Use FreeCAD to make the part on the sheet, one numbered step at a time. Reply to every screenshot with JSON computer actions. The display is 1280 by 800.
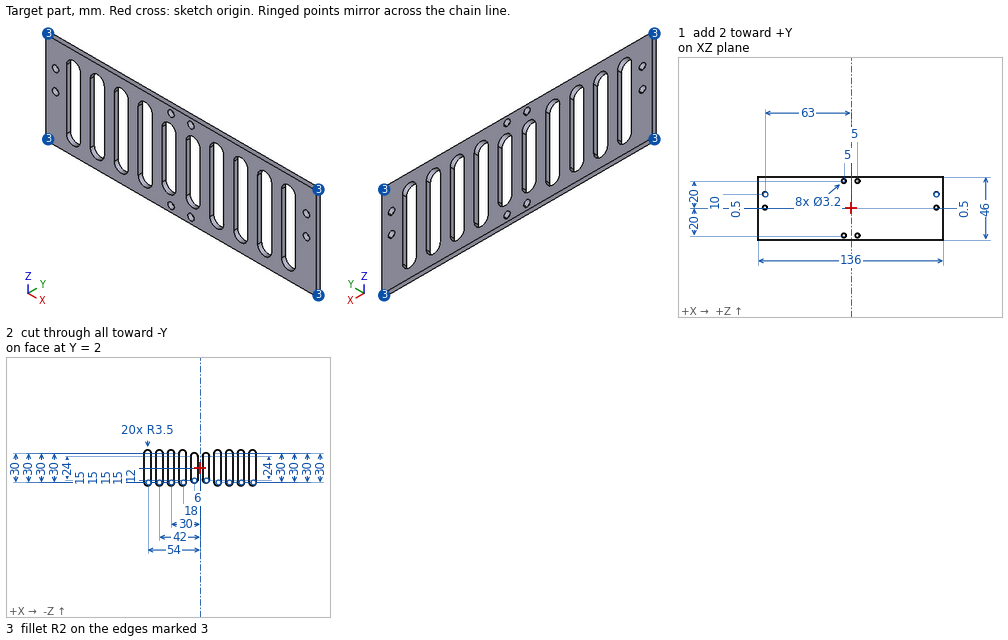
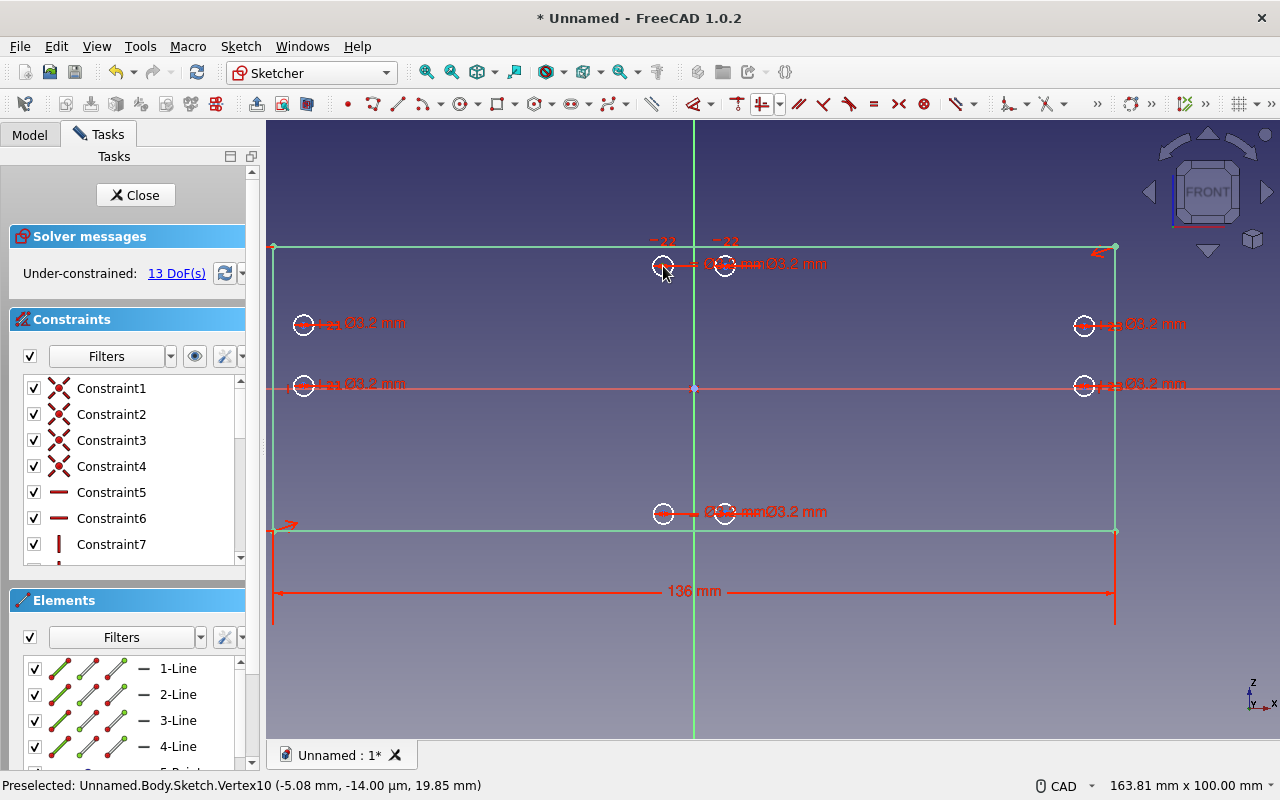
{"action": "left_click", "coordinate": [663, 514]}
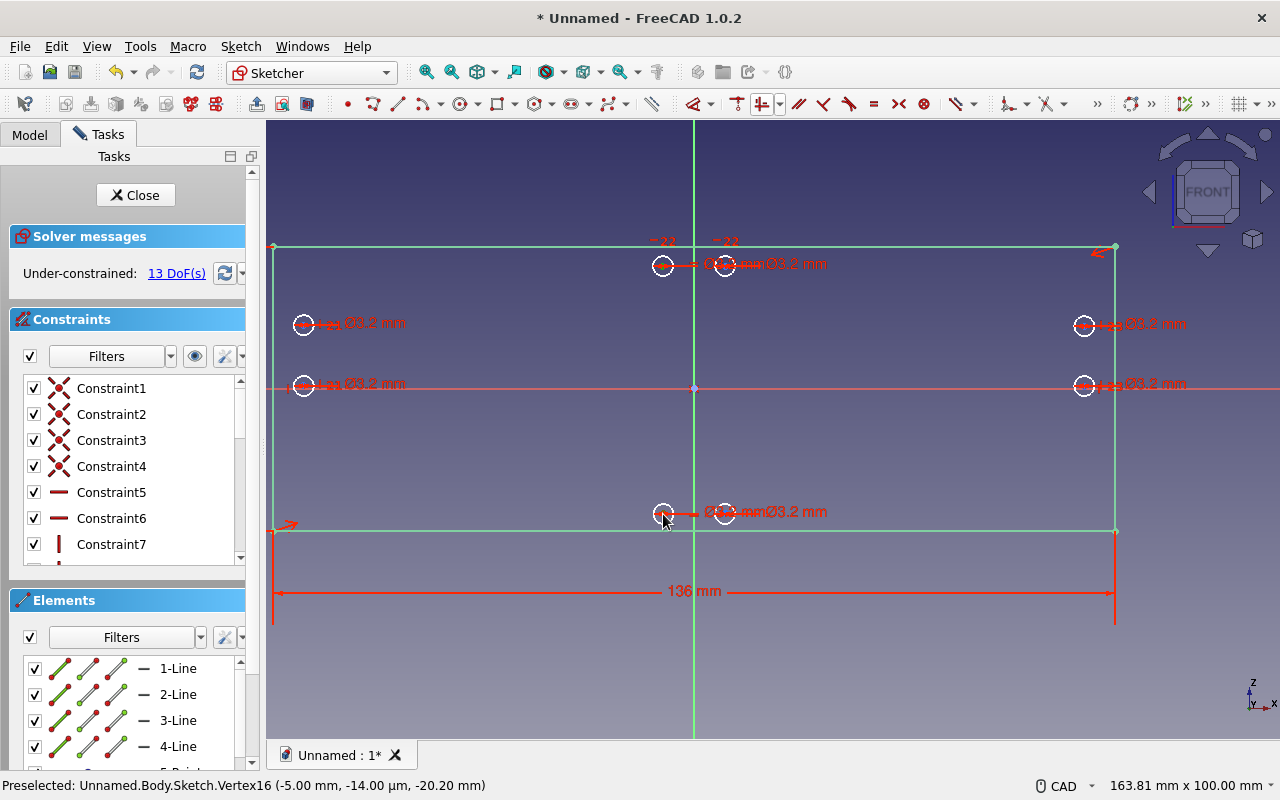
{"action": "left_click", "coordinate": [780, 104]}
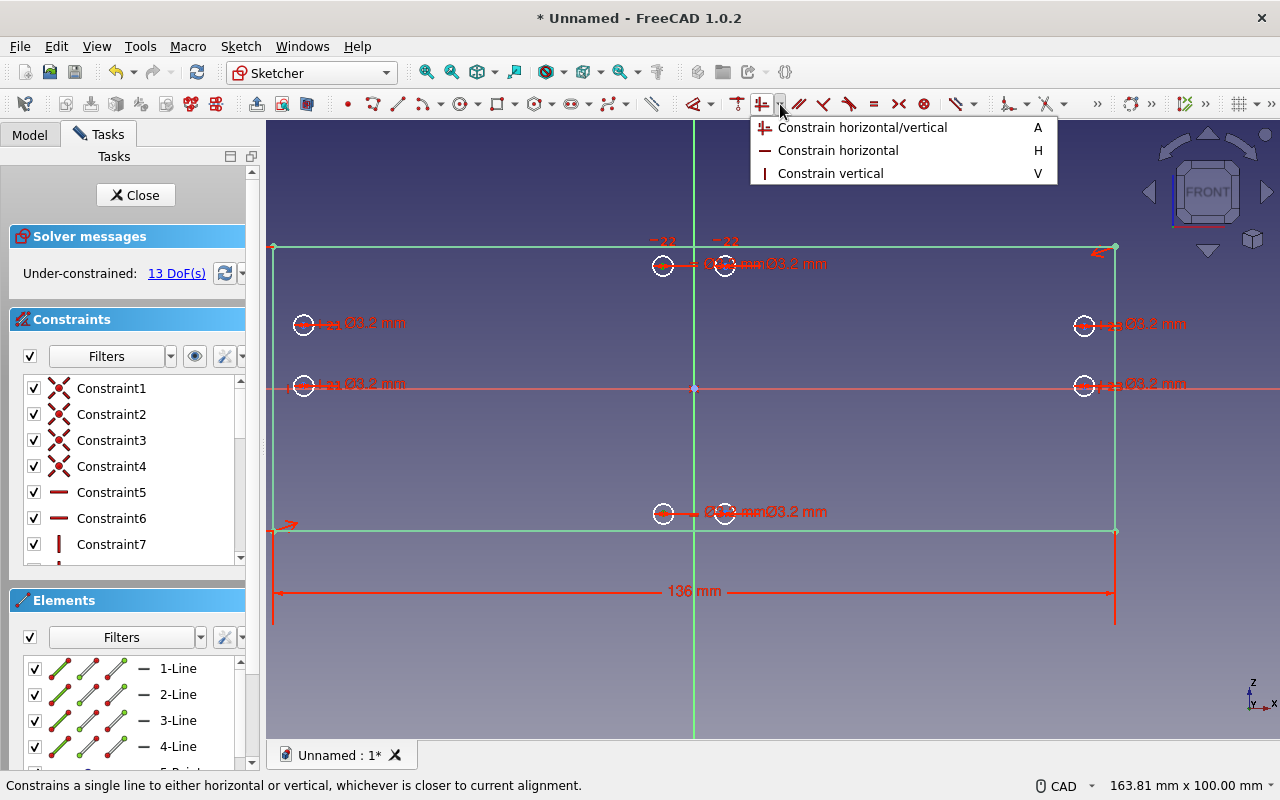
{"action": "left_click", "coordinate": [904, 174]}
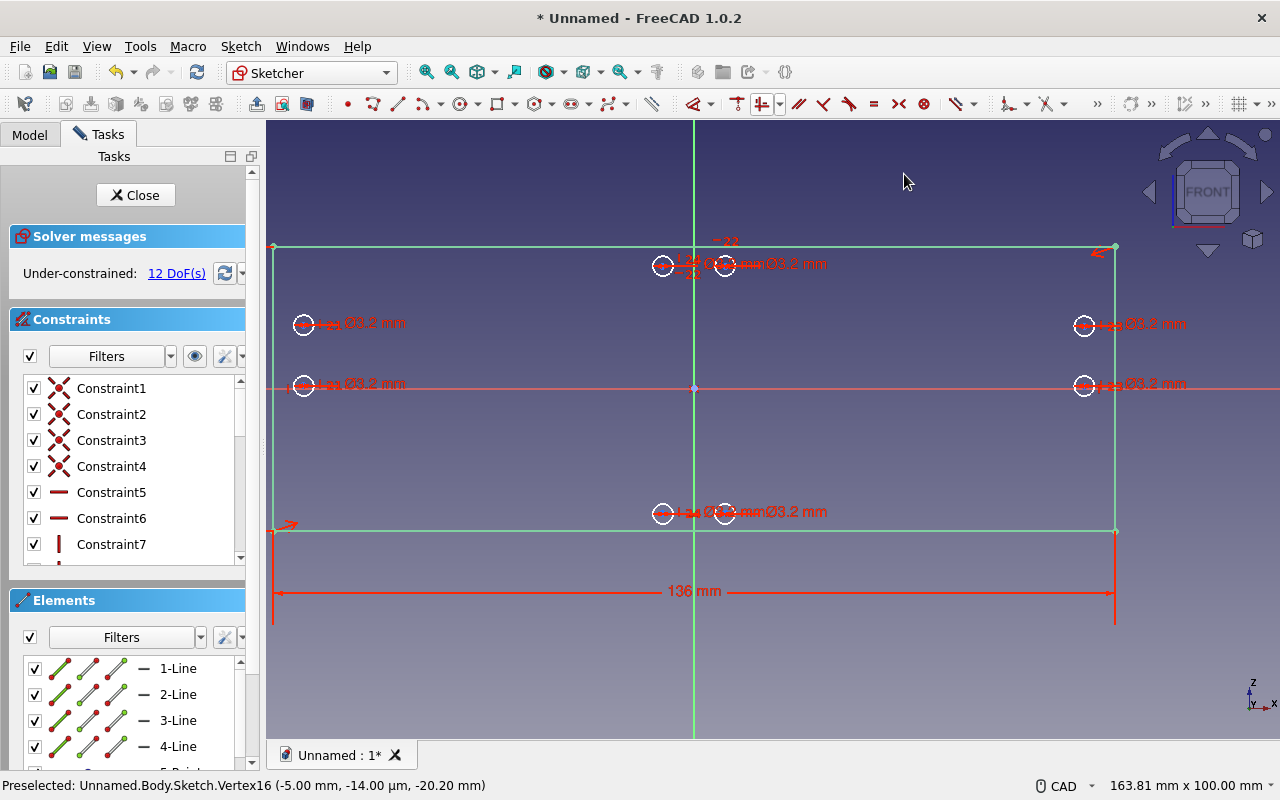
{"action": "left_click", "coordinate": [725, 266]}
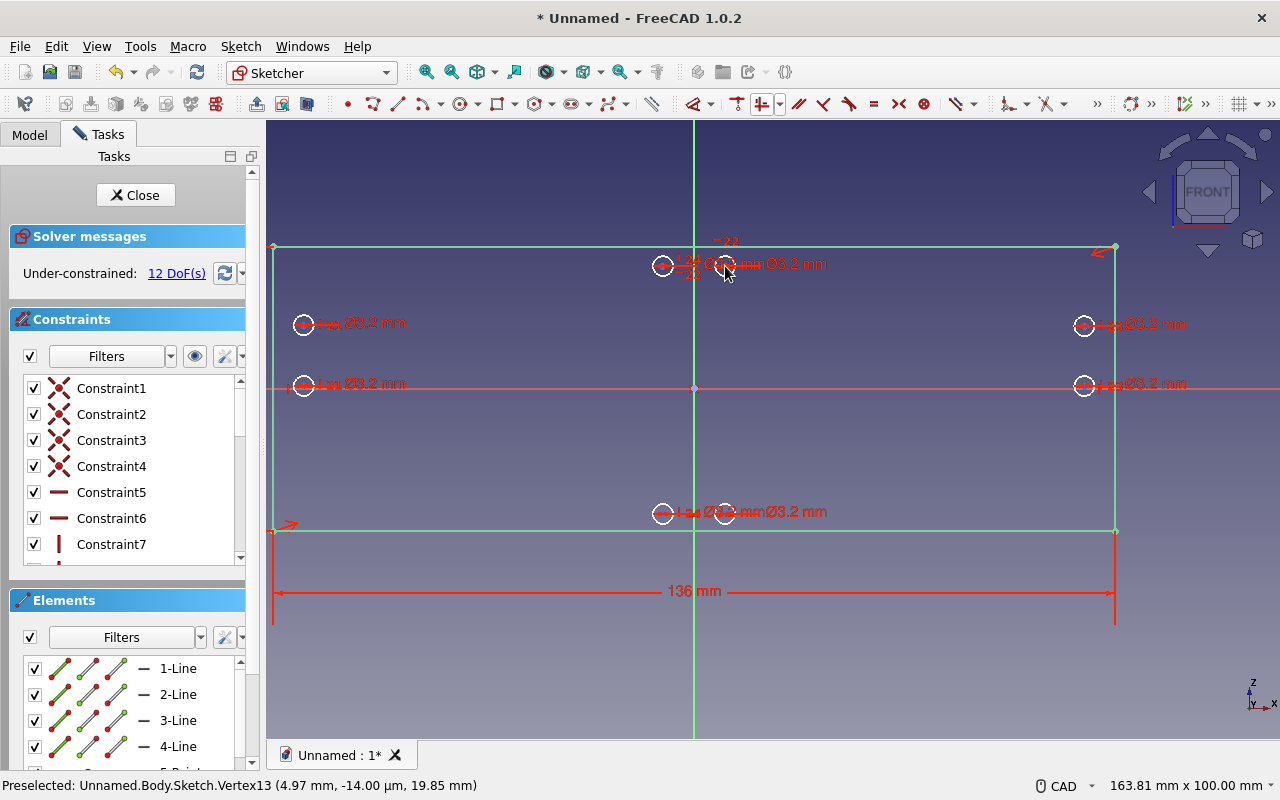
{"action": "left_click", "coordinate": [725, 514]}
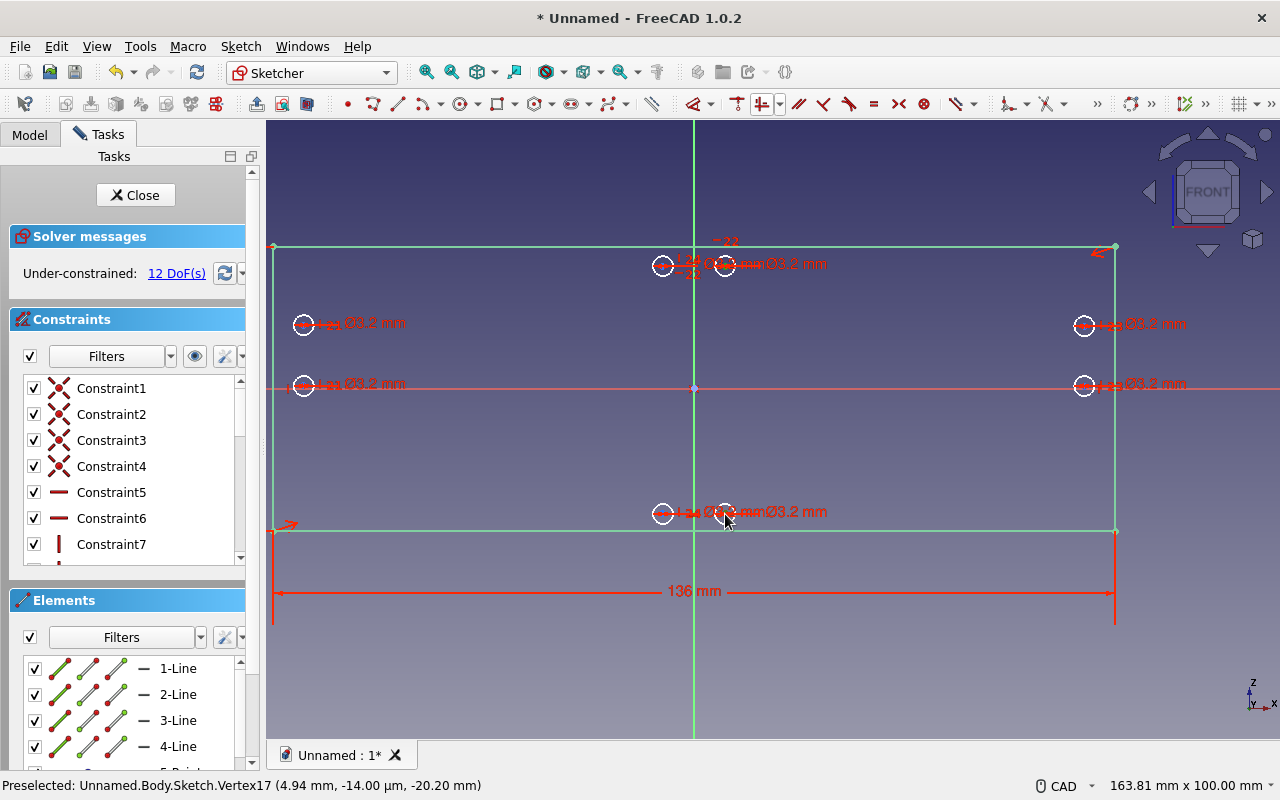
{"action": "left_click", "coordinate": [780, 104]}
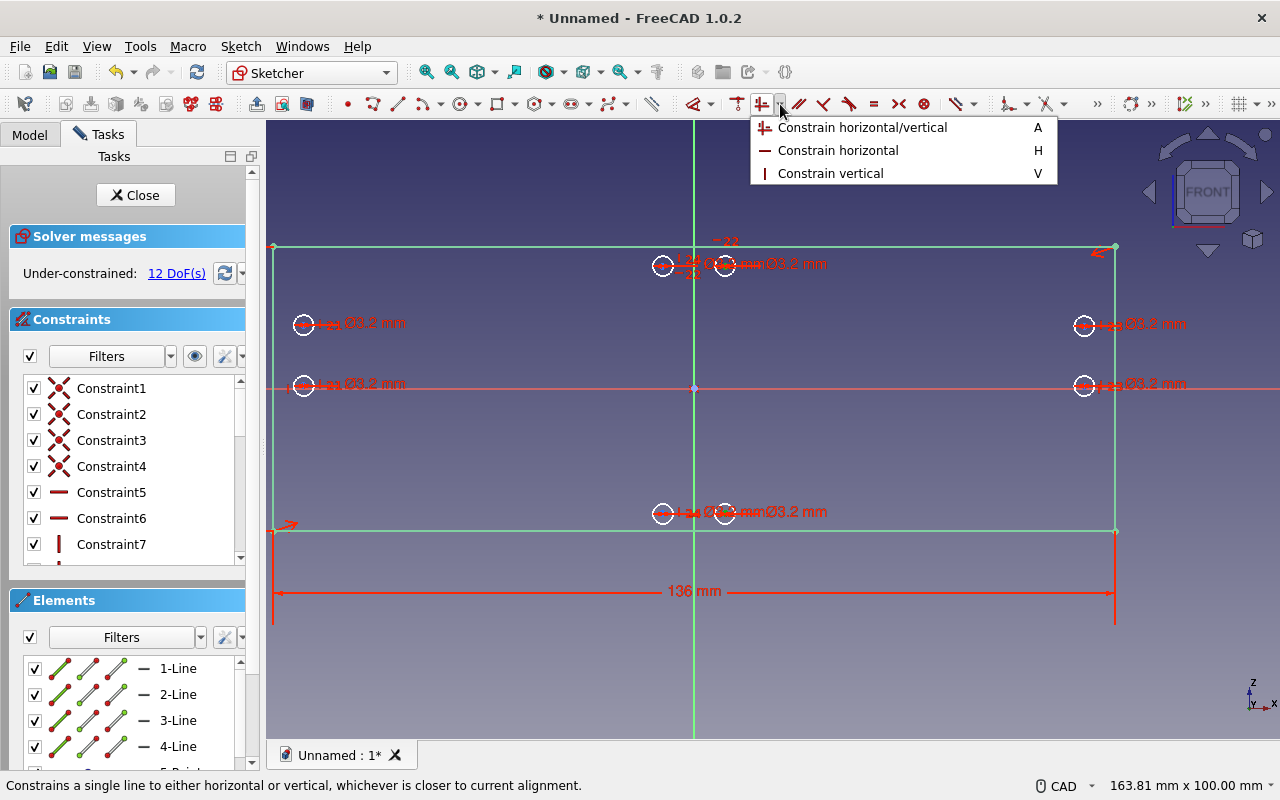
{"action": "left_click", "coordinate": [904, 174]}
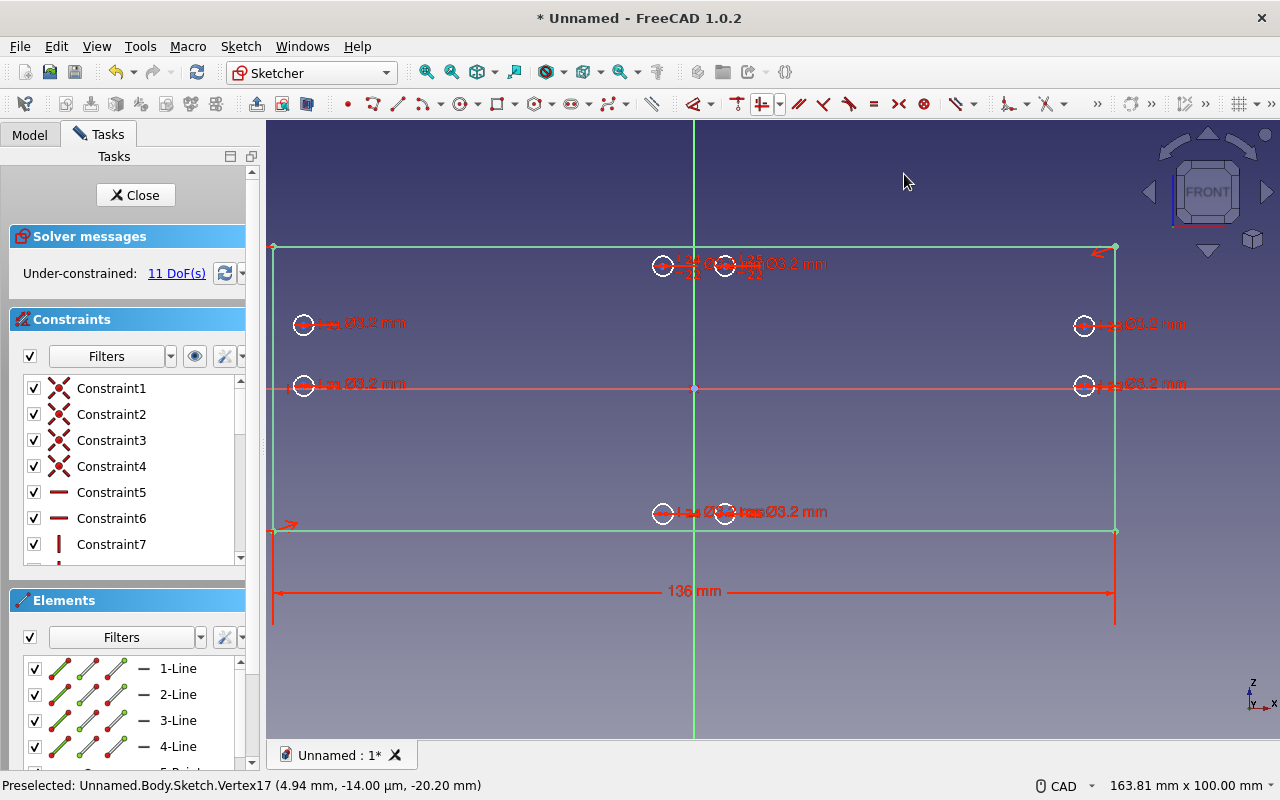
{"action": "left_click", "coordinate": [663, 514]}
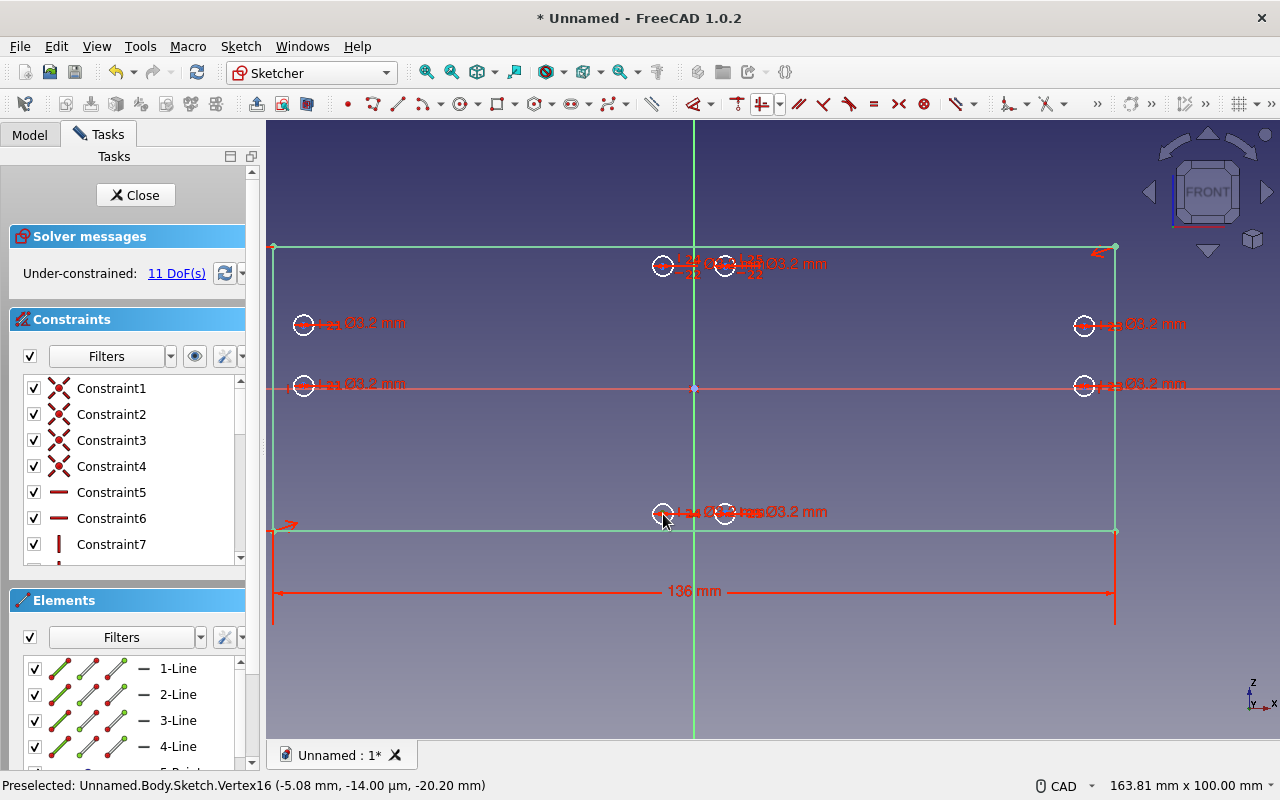
{"action": "left_click", "coordinate": [725, 514]}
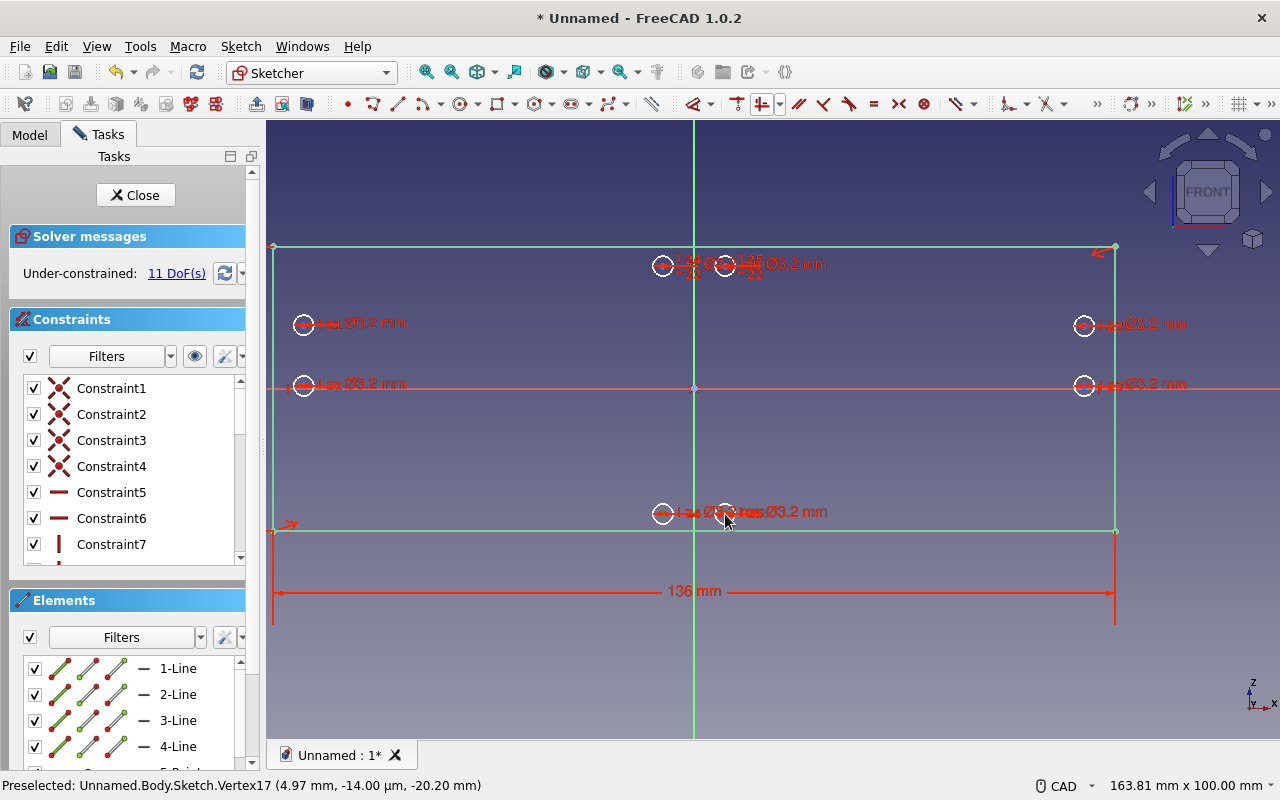
{"action": "key", "text": "h"}